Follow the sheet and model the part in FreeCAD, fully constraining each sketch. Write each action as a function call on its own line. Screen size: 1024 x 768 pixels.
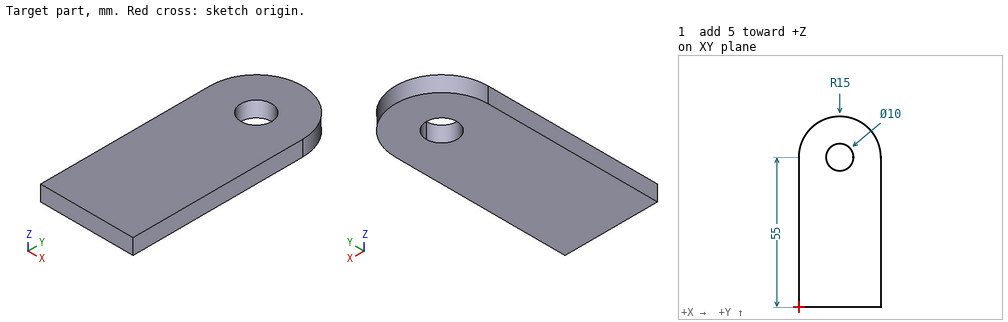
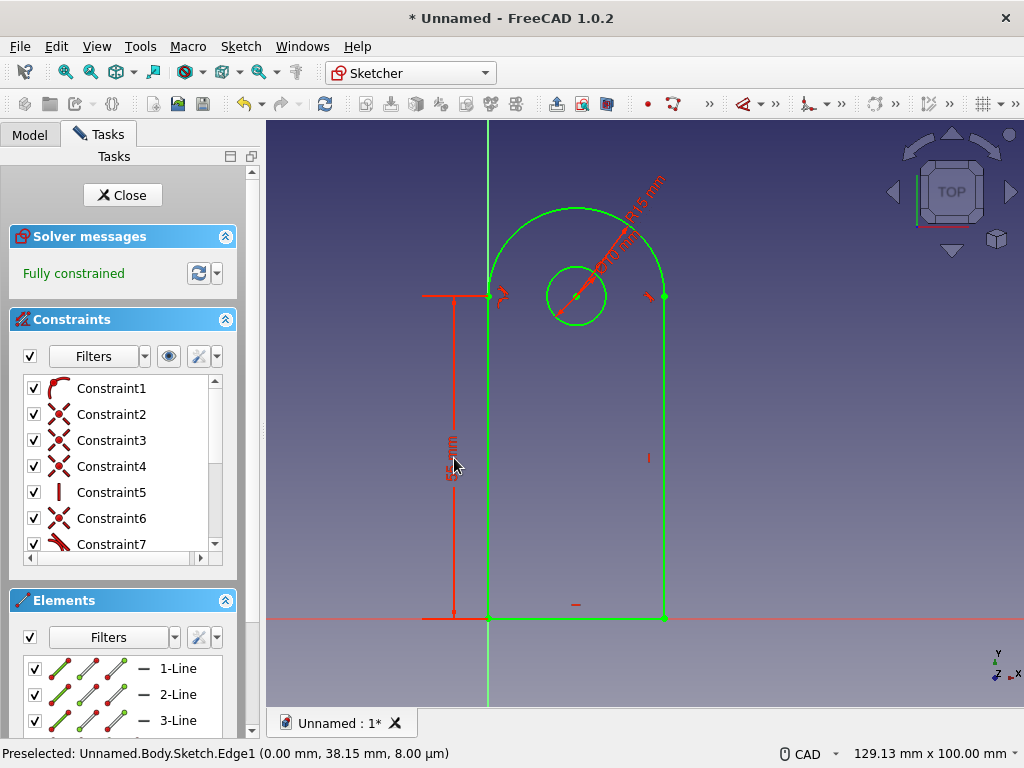
click(123, 195)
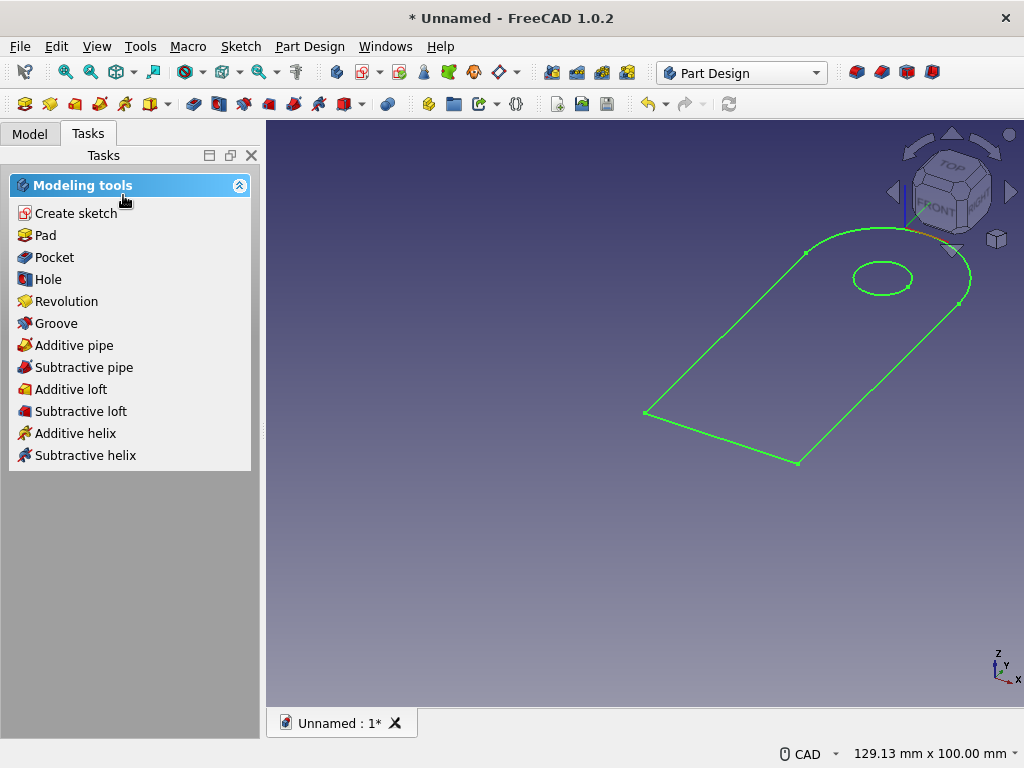
click(25, 104)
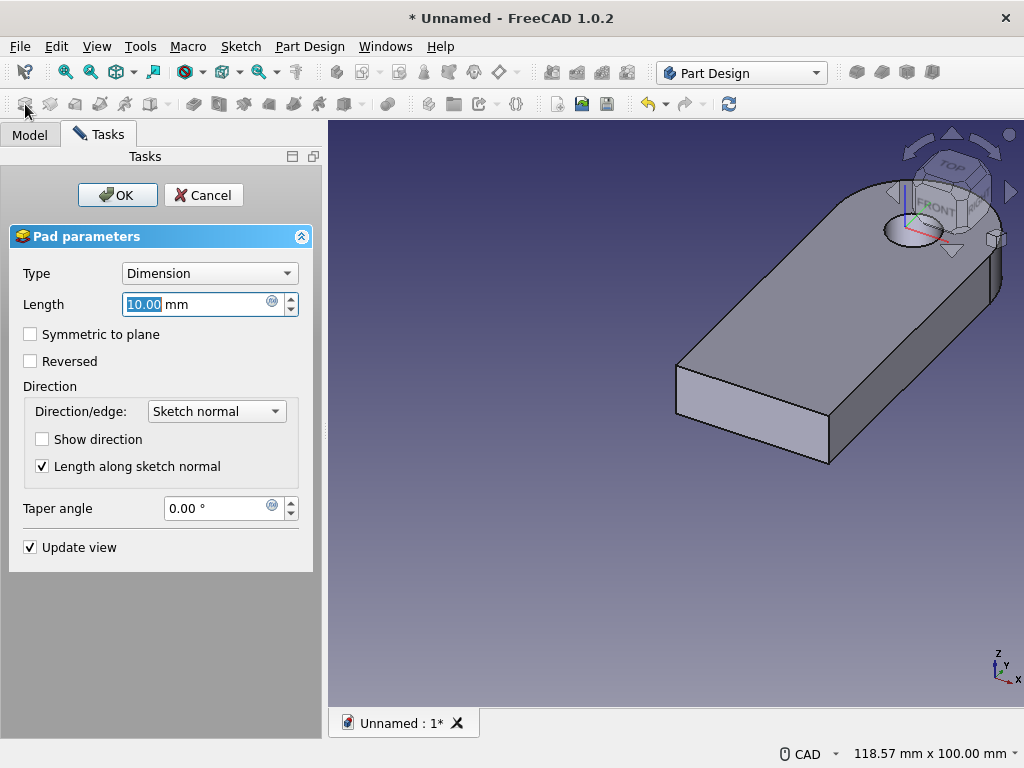
text(5)
key(Tab)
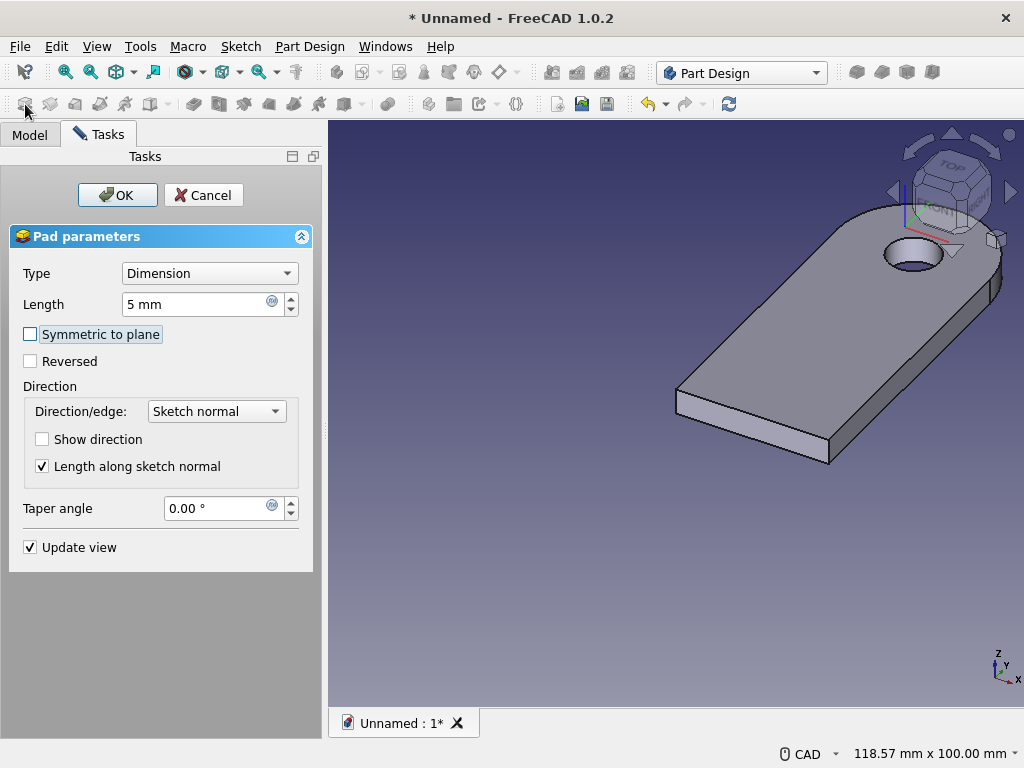
click(118, 195)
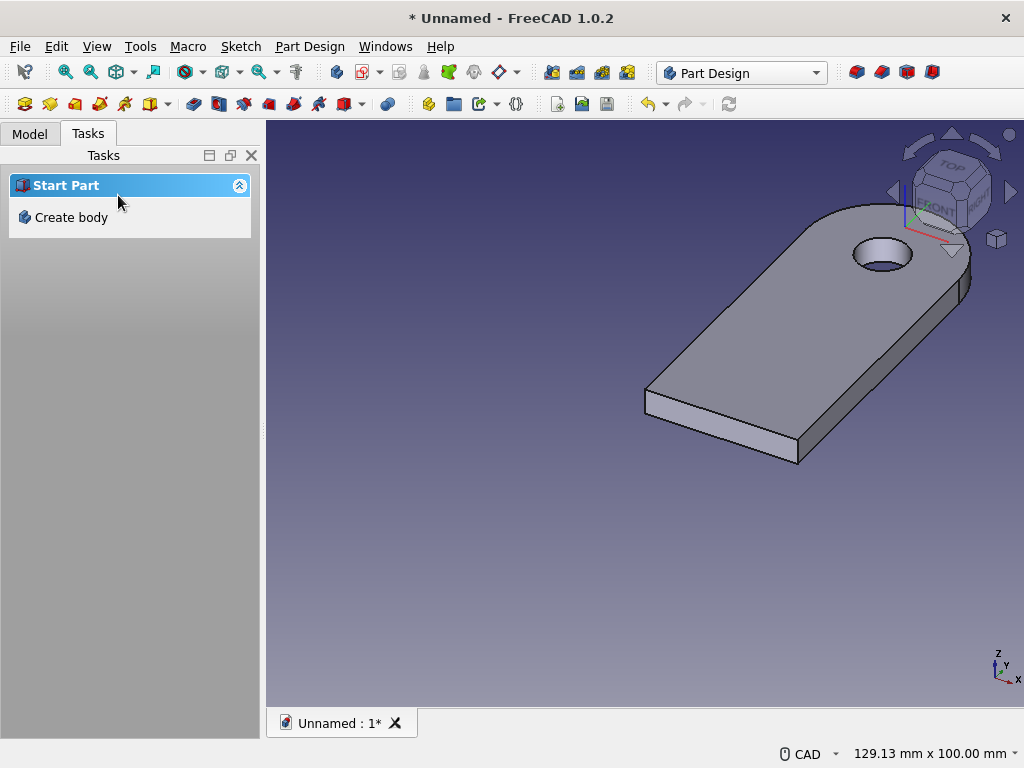
key(0)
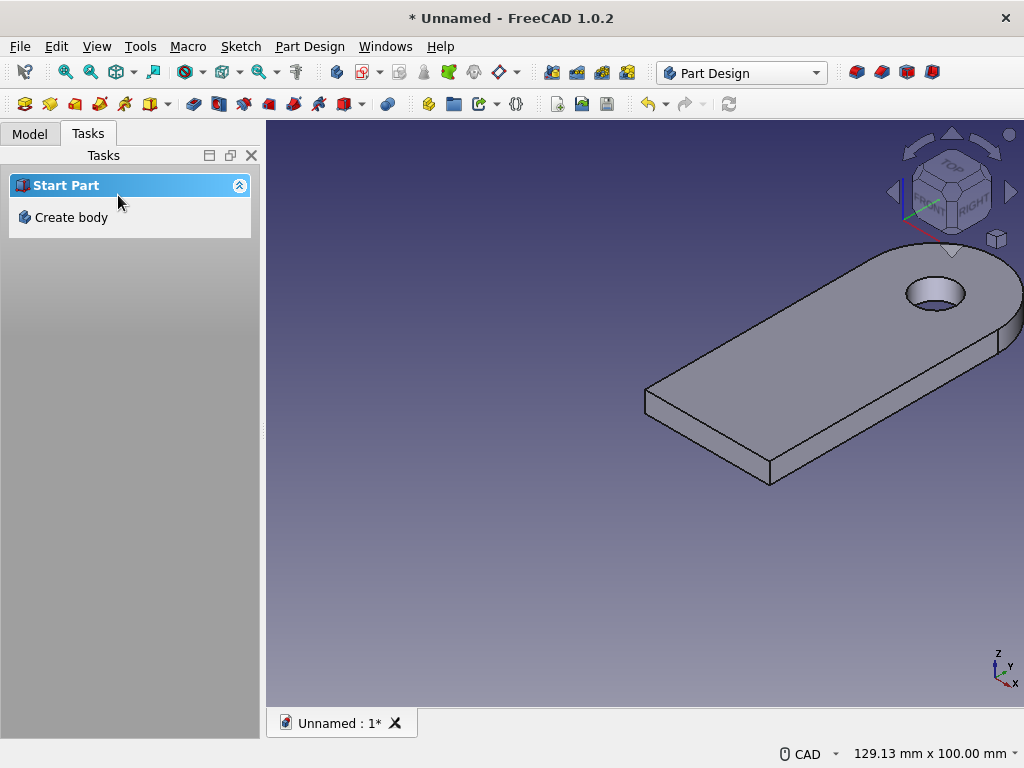
key(v)
key(f)